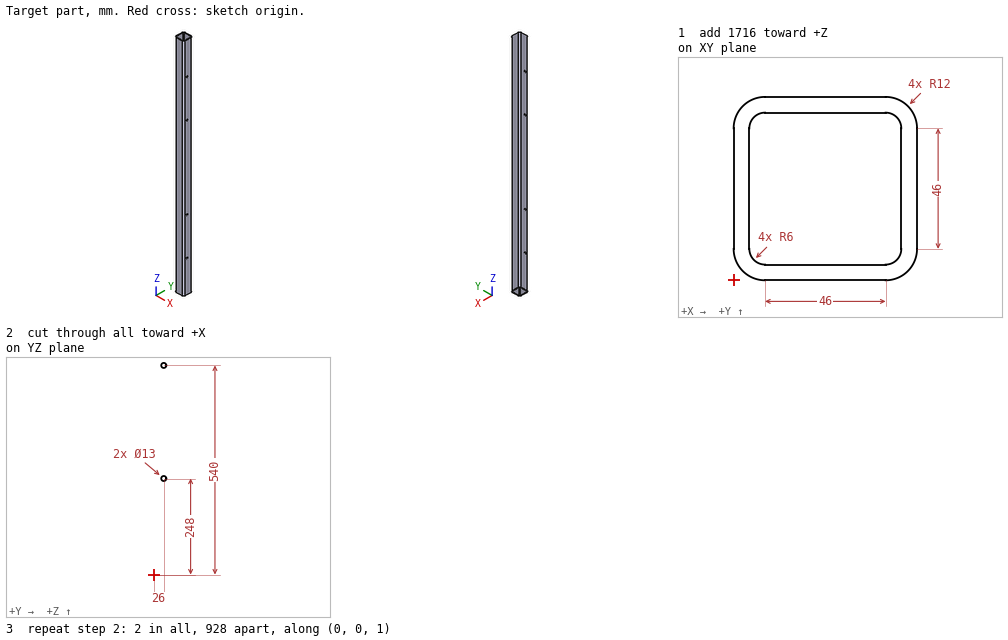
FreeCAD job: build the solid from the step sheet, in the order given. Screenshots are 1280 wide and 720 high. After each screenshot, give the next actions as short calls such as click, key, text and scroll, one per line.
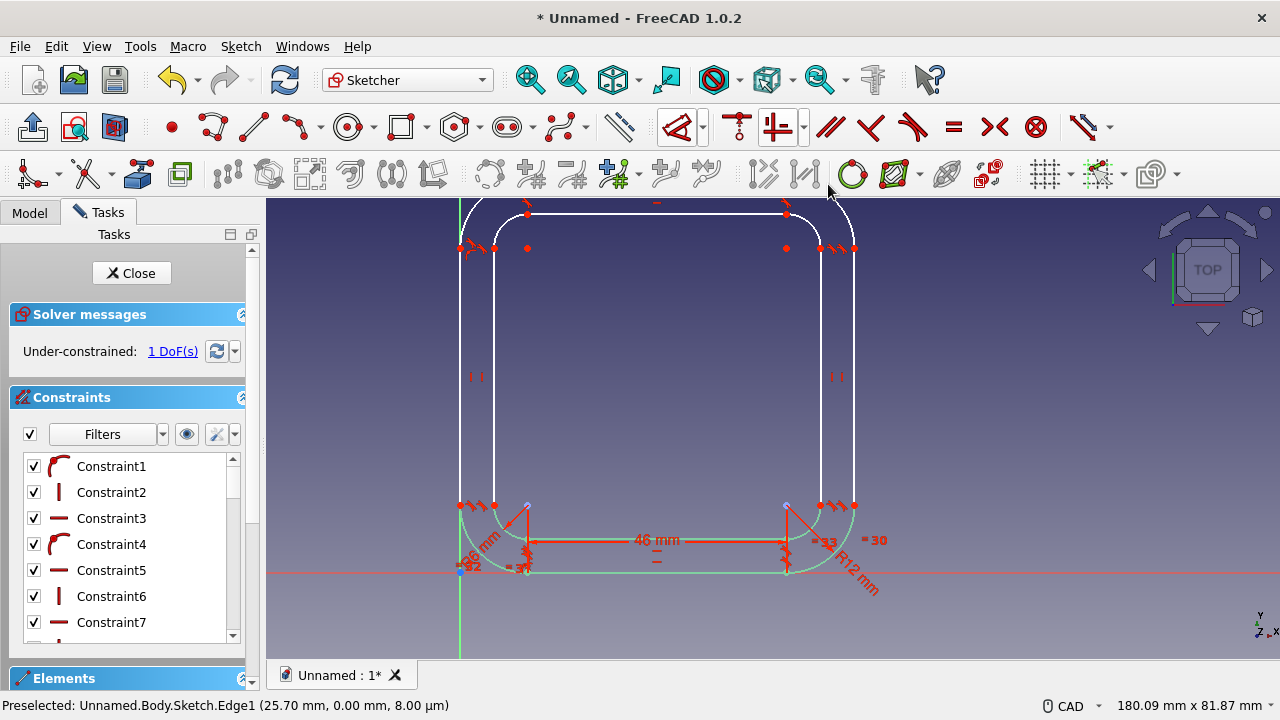
click(854, 428)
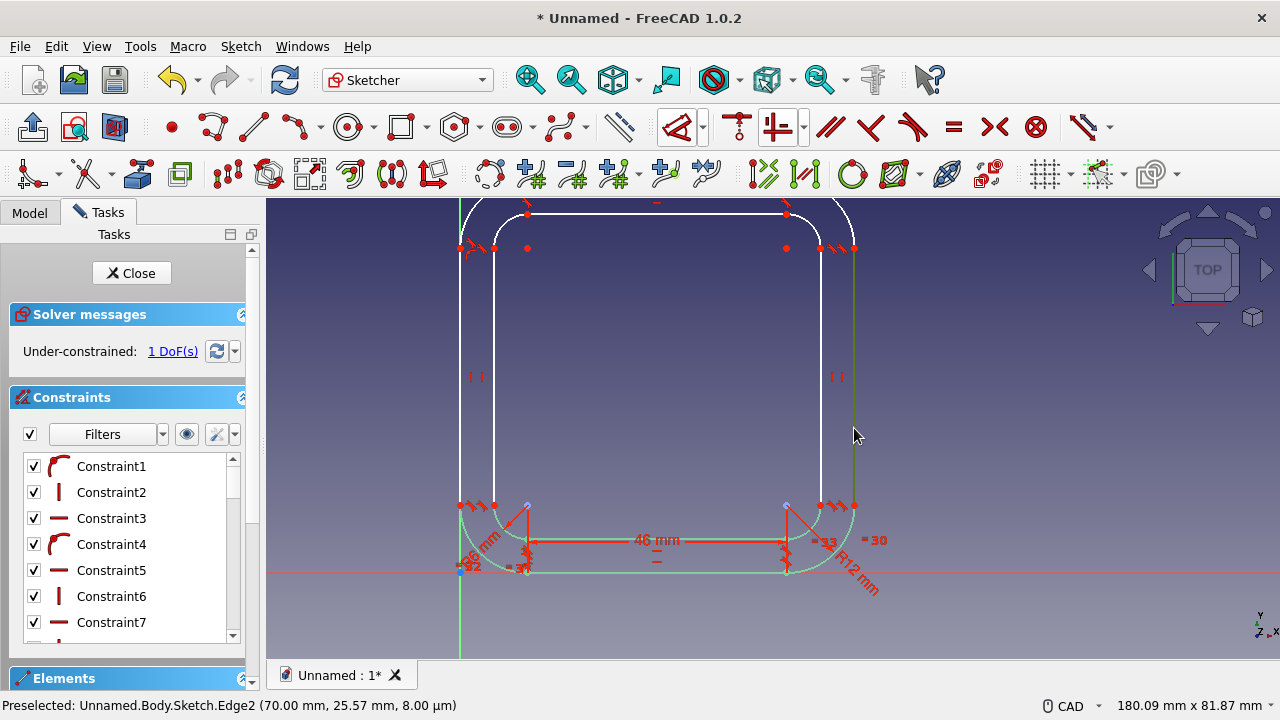
click(702, 128)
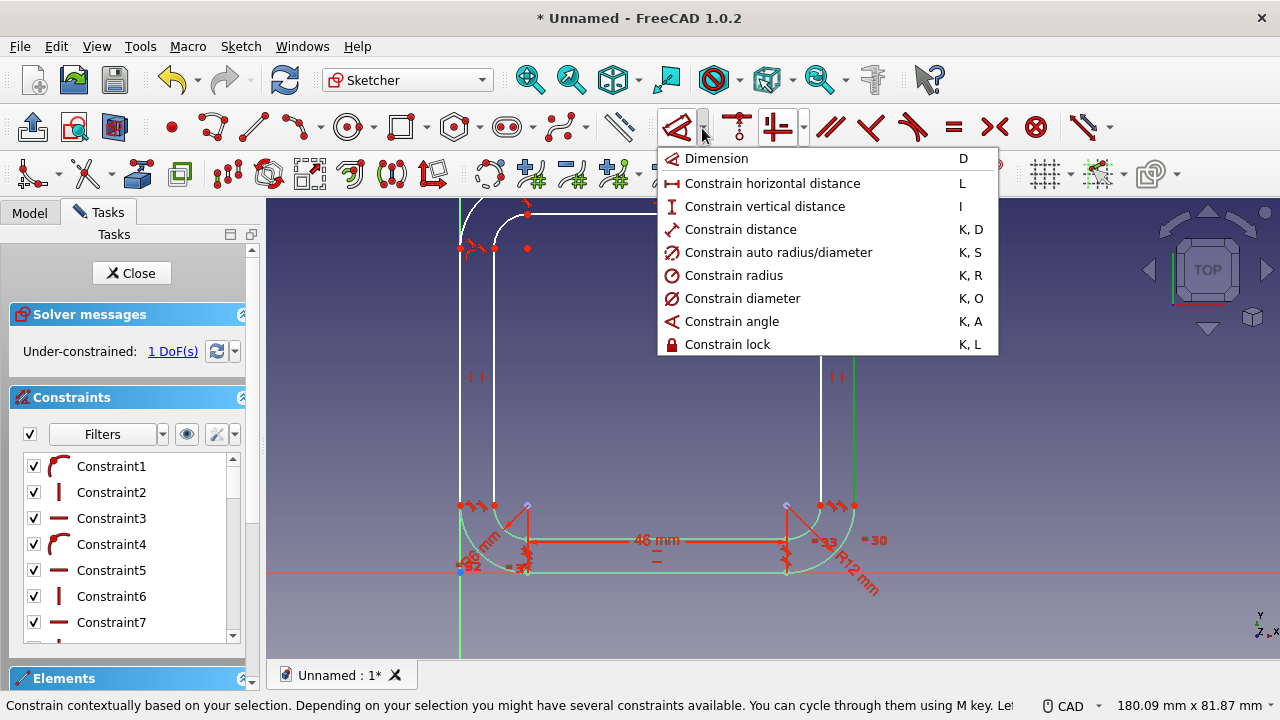
click(828, 206)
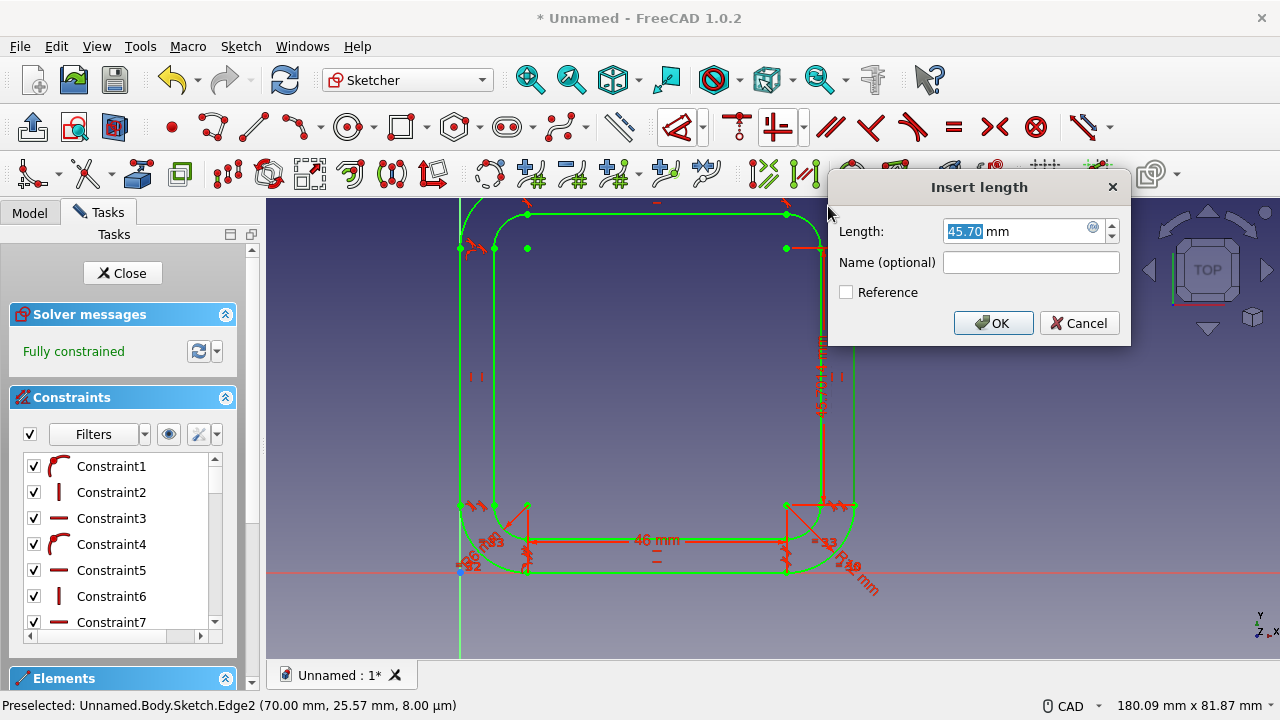
text(46)
key(Return)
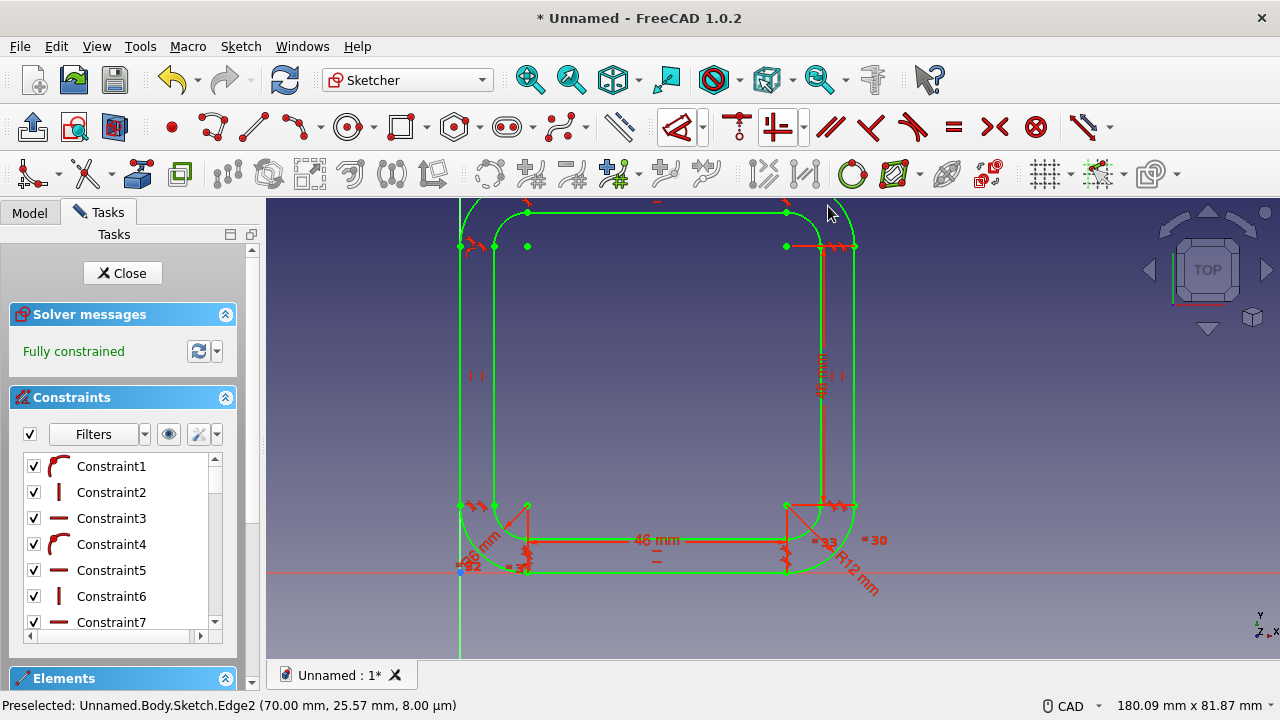
click(123, 273)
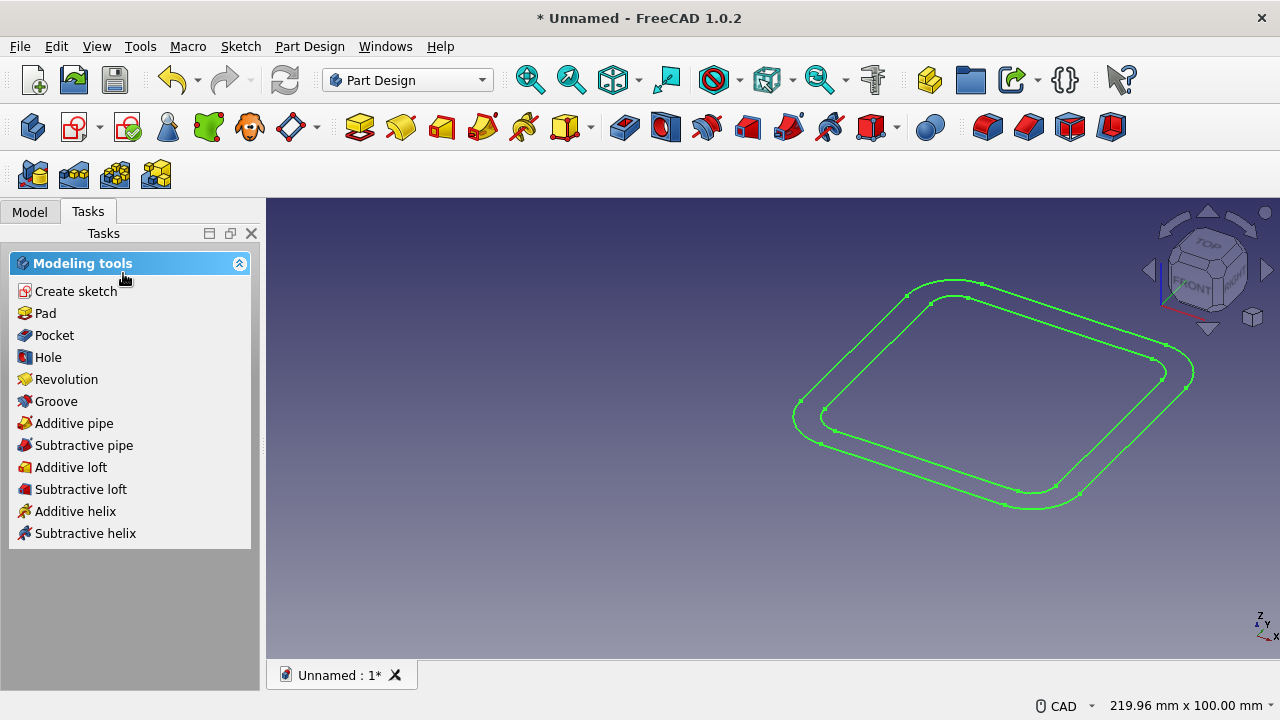
click(360, 128)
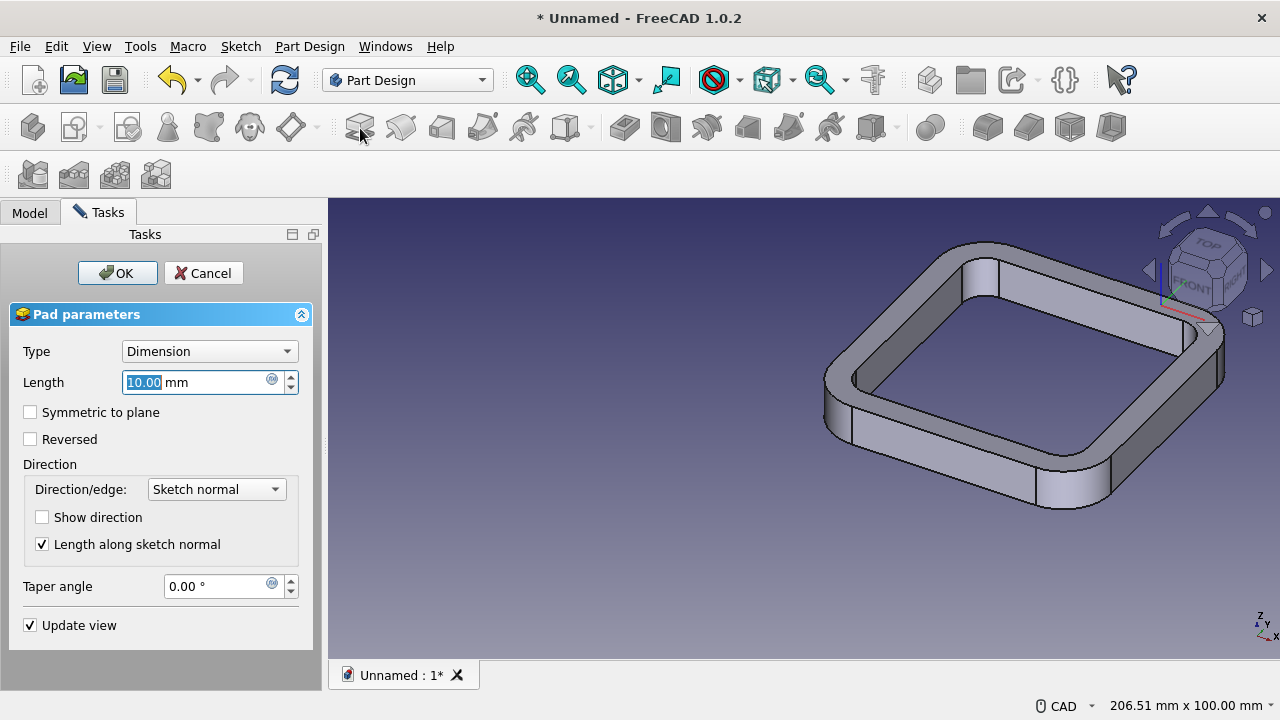
text(1716)
key(Tab)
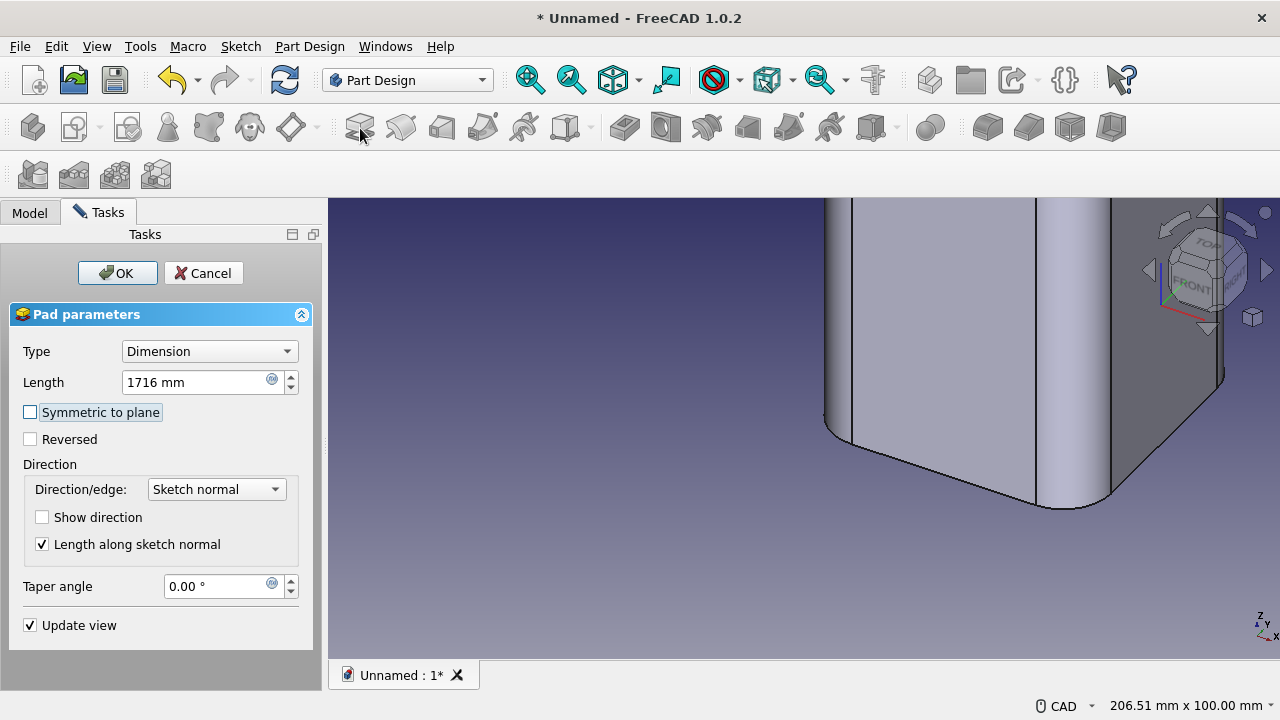
click(118, 273)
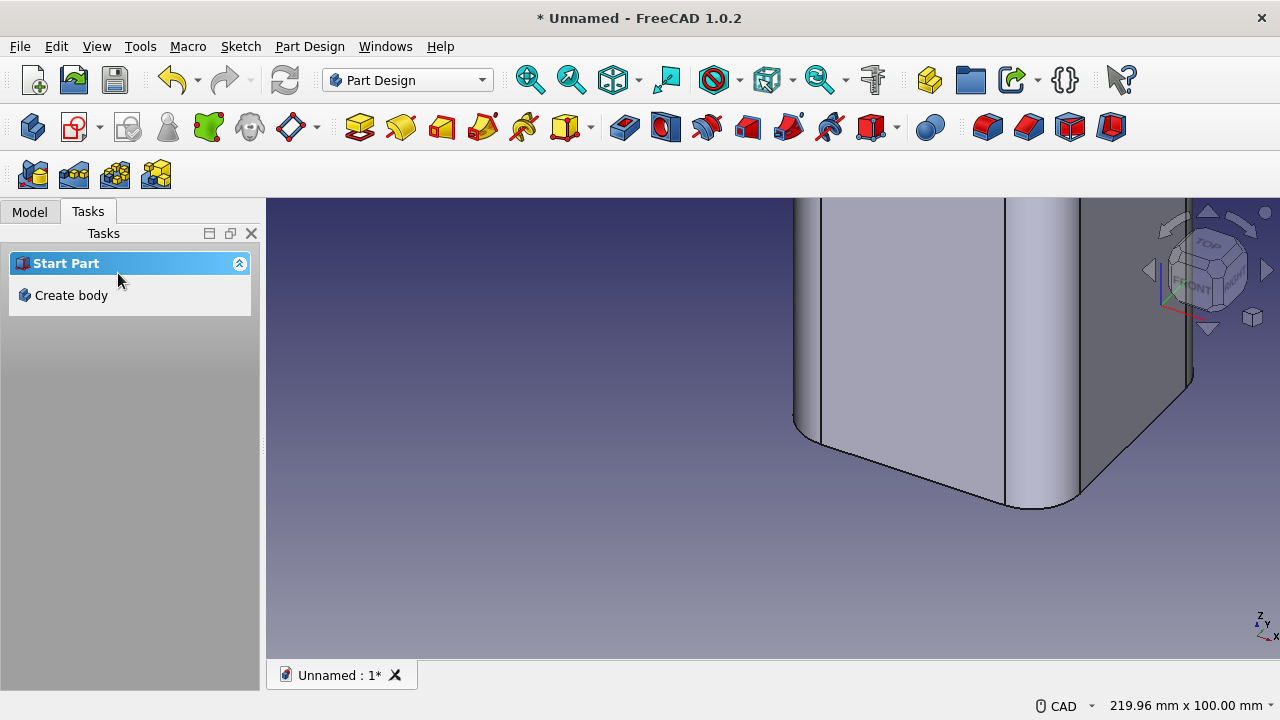
click(531, 80)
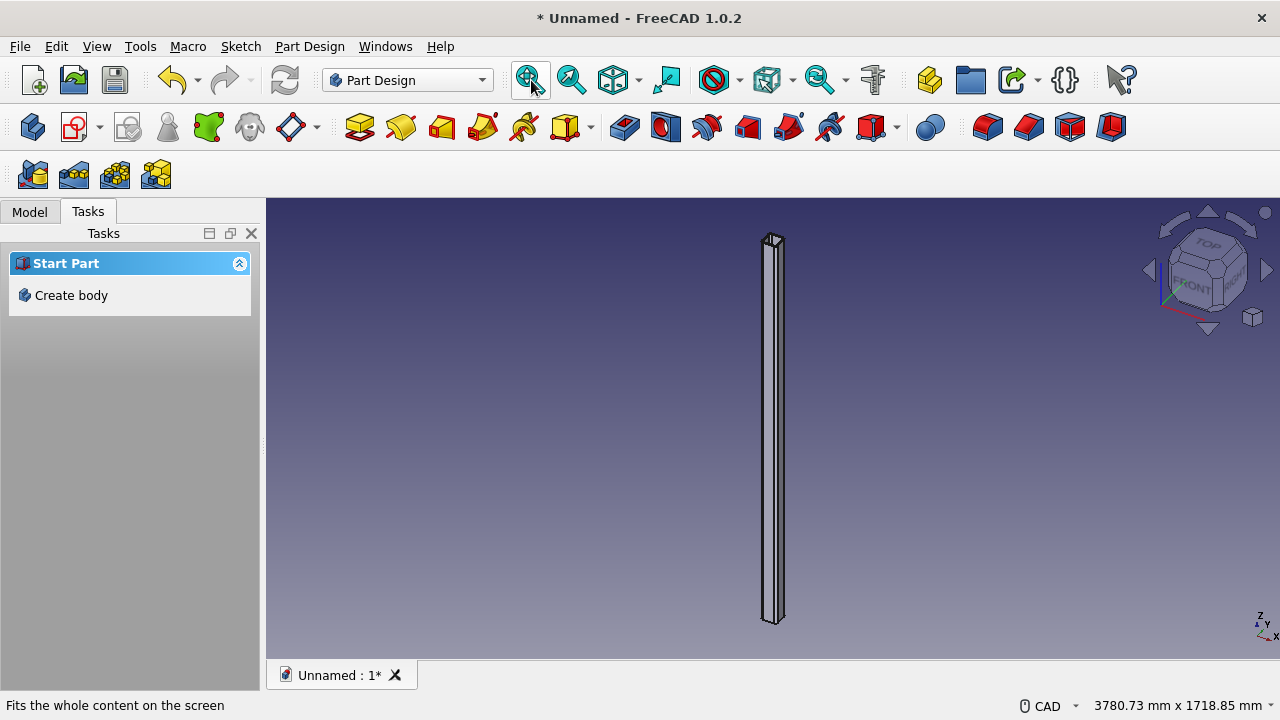
click(74, 128)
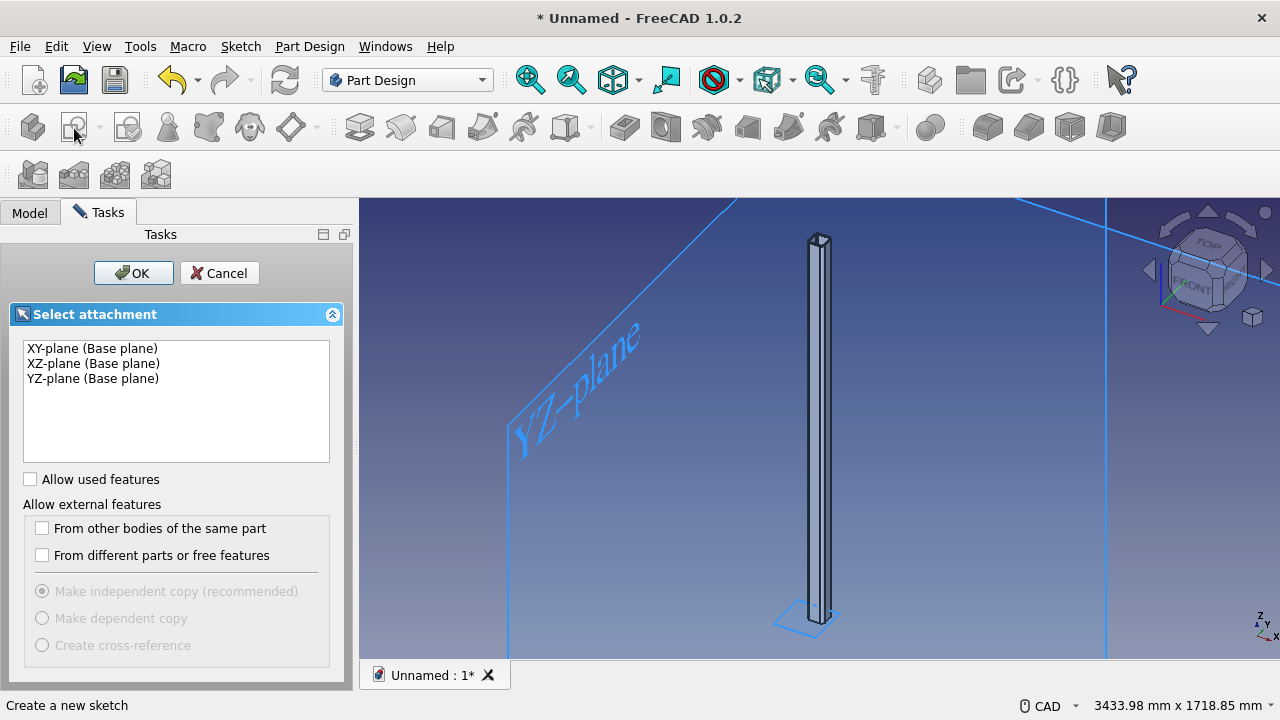
click(84, 378)